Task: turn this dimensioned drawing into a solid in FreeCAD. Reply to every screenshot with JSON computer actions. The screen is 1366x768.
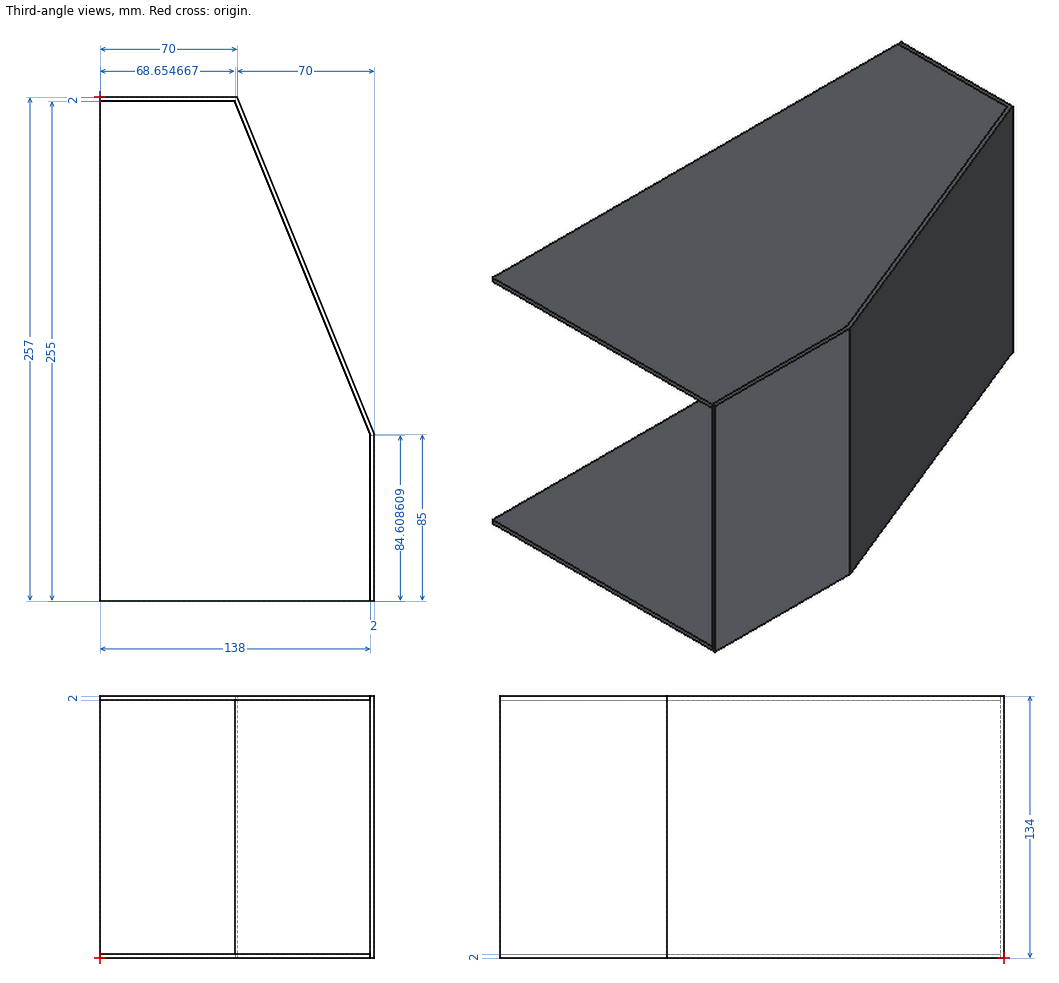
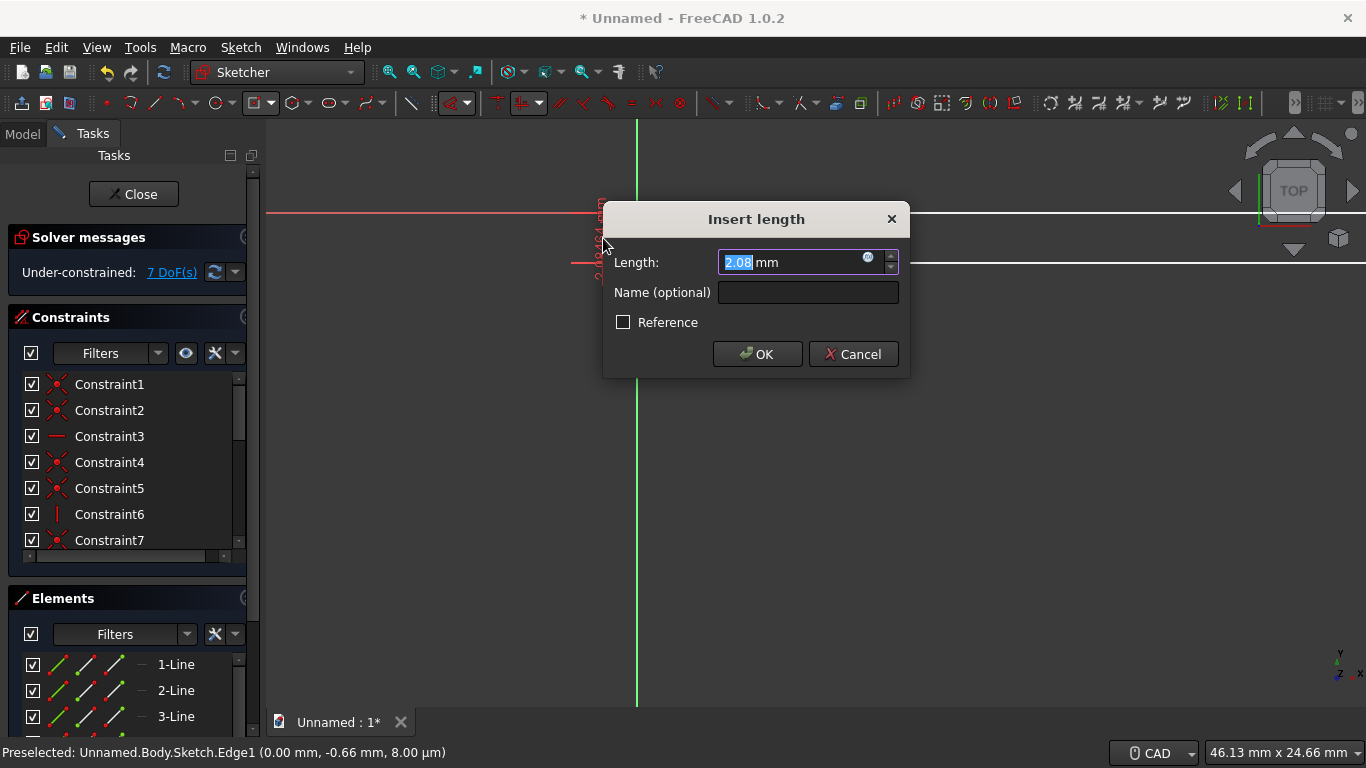
{"action": "type", "text": "2"}
{"action": "key", "text": "Return"}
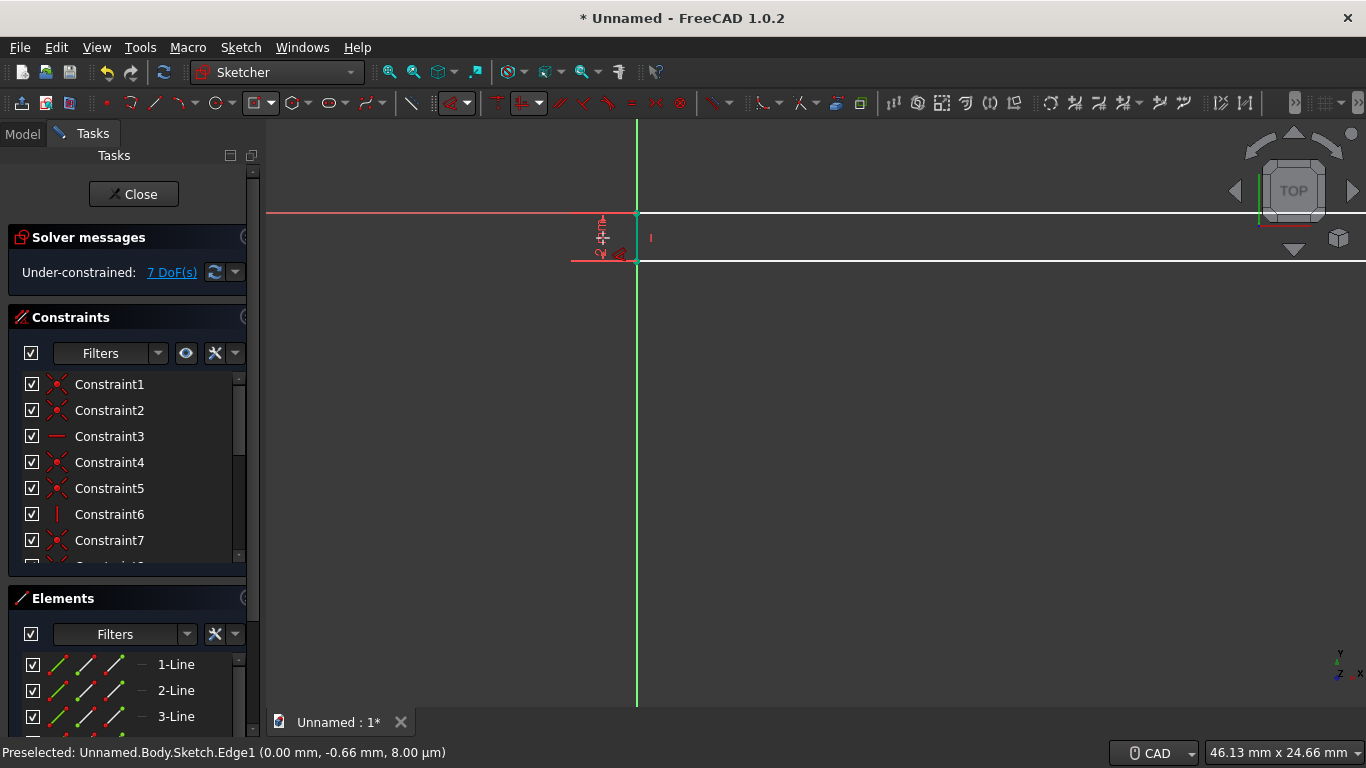
{"action": "scroll", "coordinate": [647, 228], "scroll_direction": "down", "scroll_amount": 14}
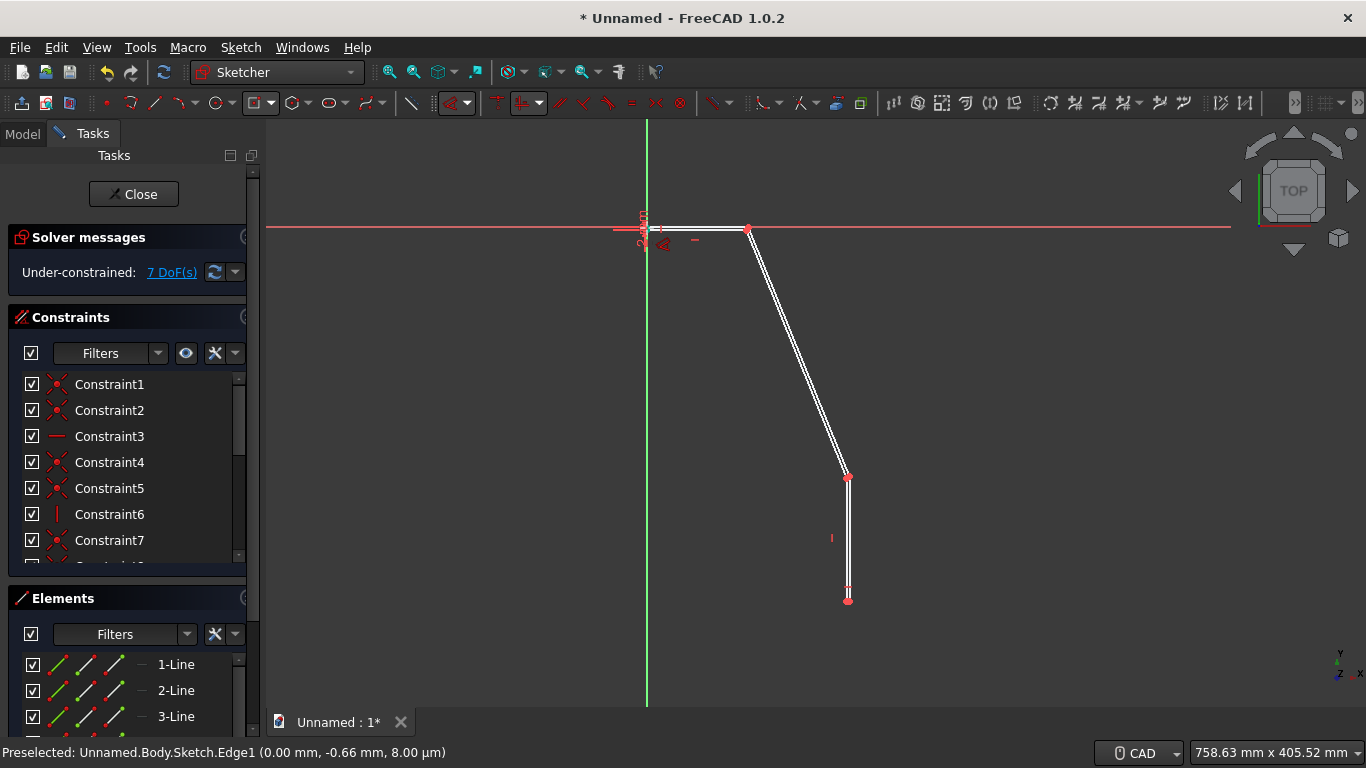
{"action": "scroll", "coordinate": [848, 601], "scroll_direction": "up", "scroll_amount": 14}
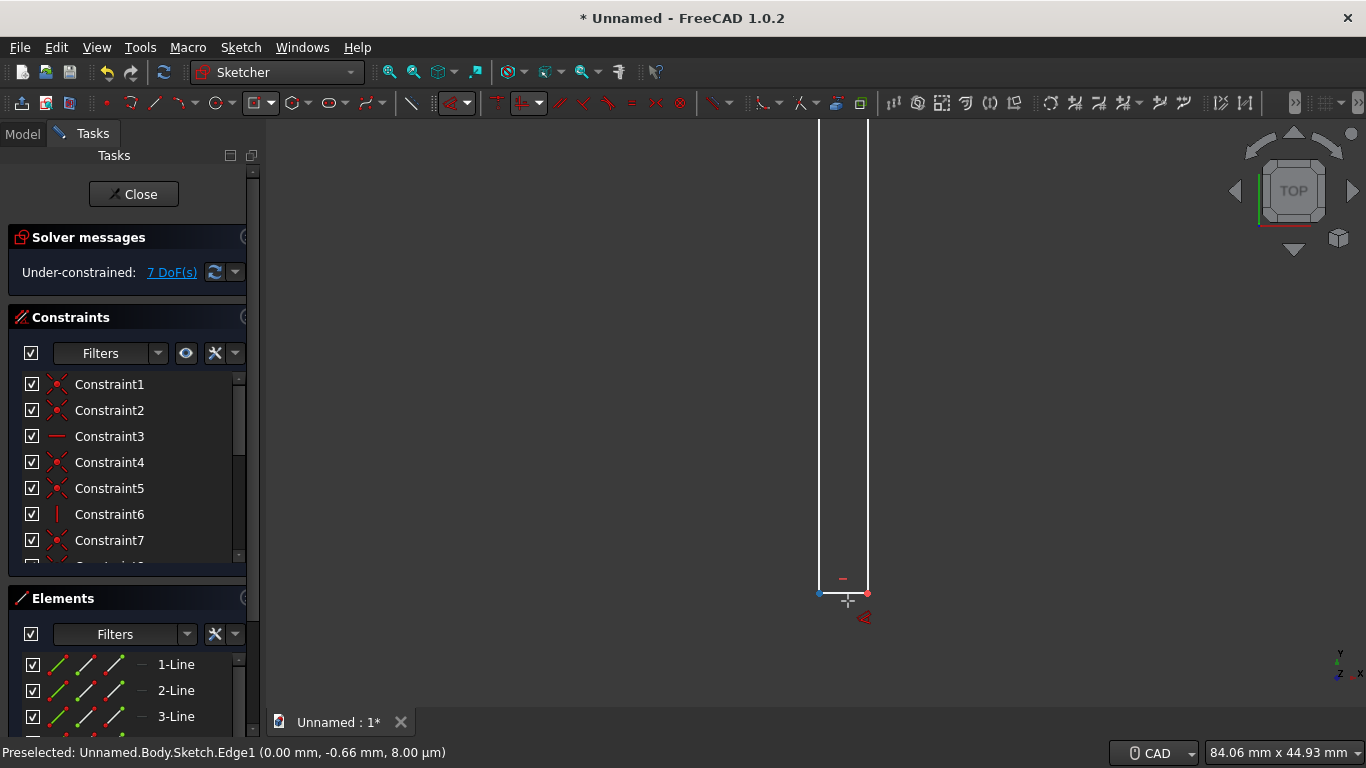
{"action": "left_click", "coordinate": [834, 593]}
{"action": "left_click", "coordinate": [843, 627]}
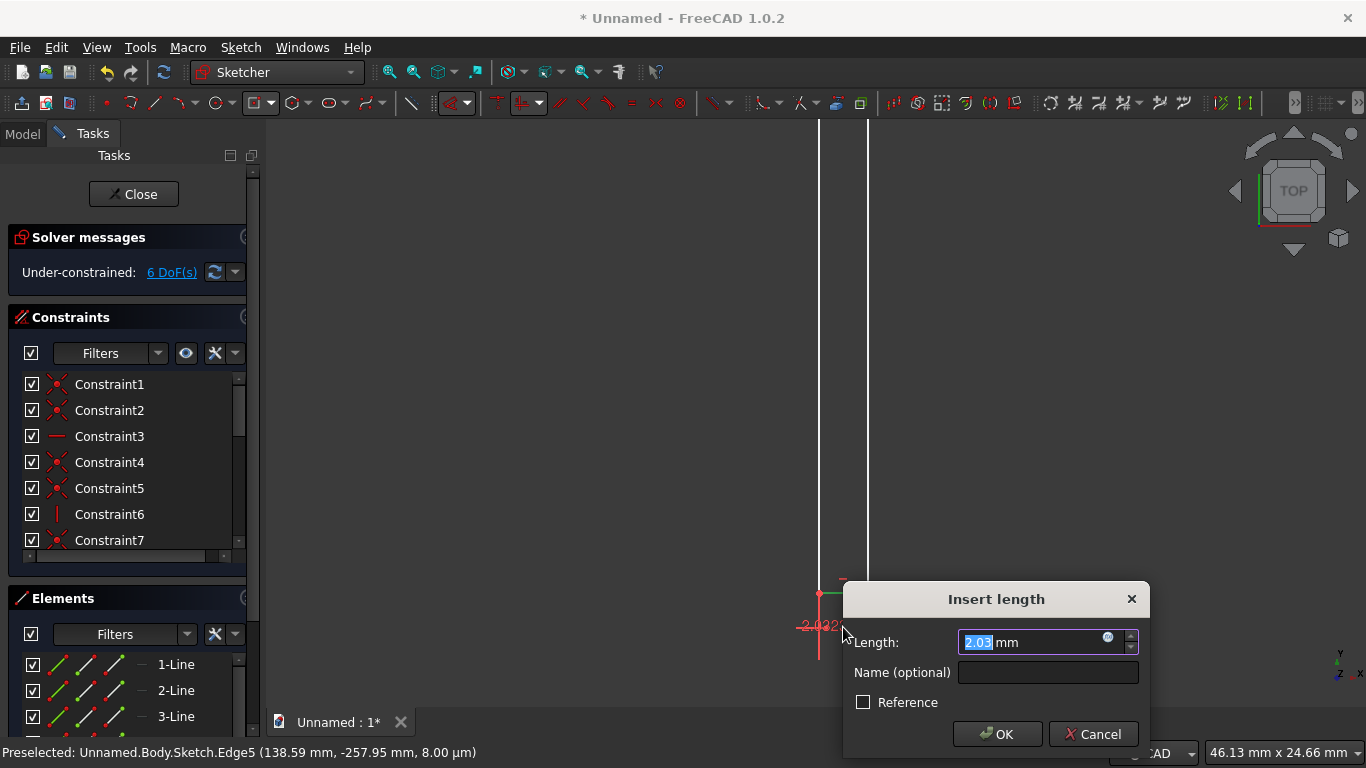
{"action": "type", "text": "2"}
{"action": "key", "text": "Return"}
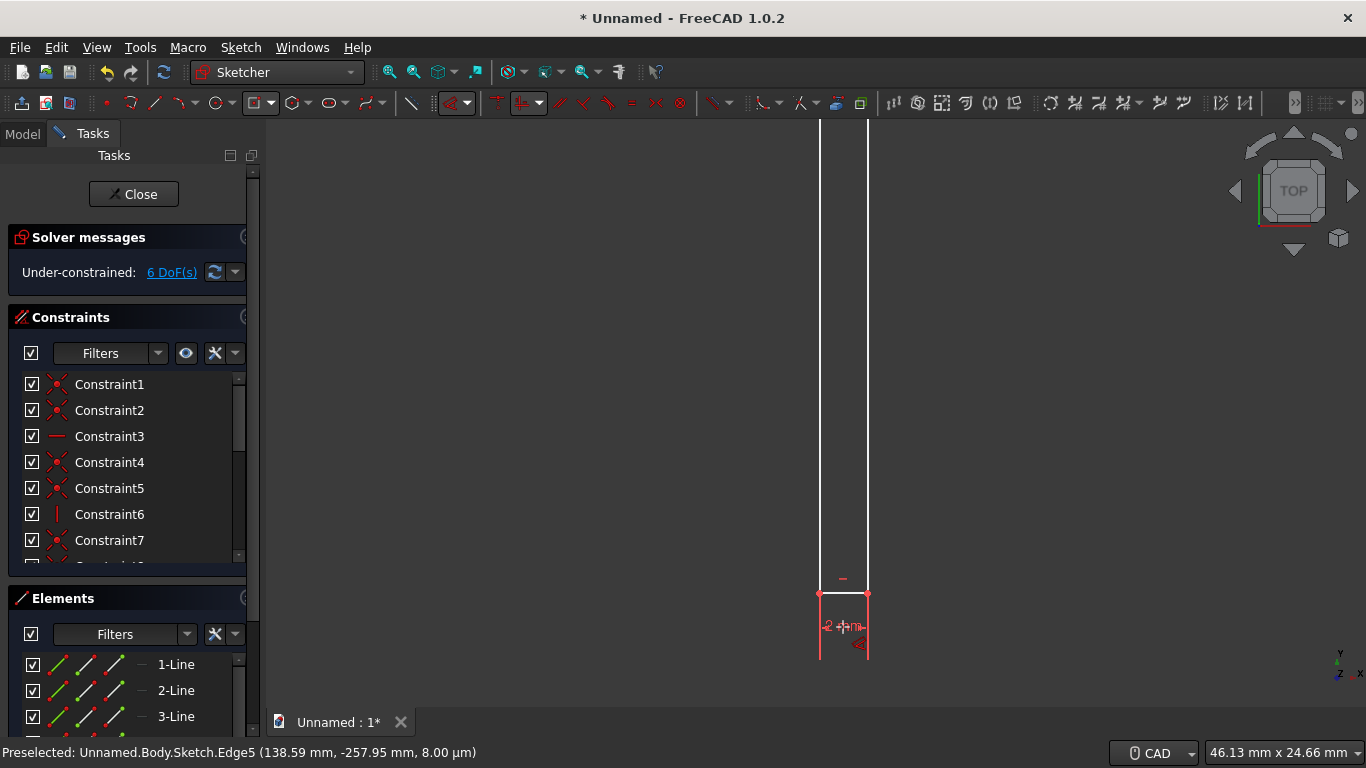
{"action": "scroll", "coordinate": [848, 601], "scroll_direction": "down", "scroll_amount": 14}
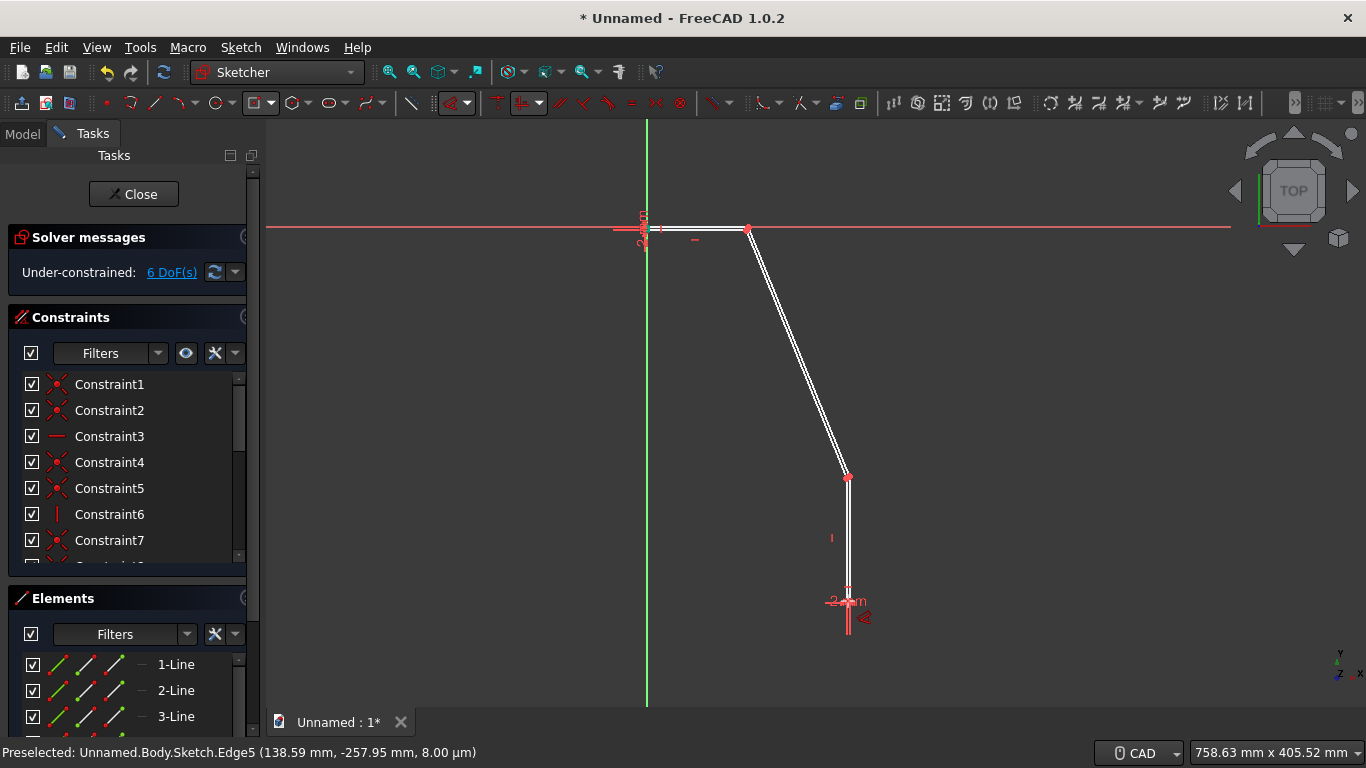
{"action": "scroll", "coordinate": [850, 576], "scroll_direction": "up", "scroll_amount": 8}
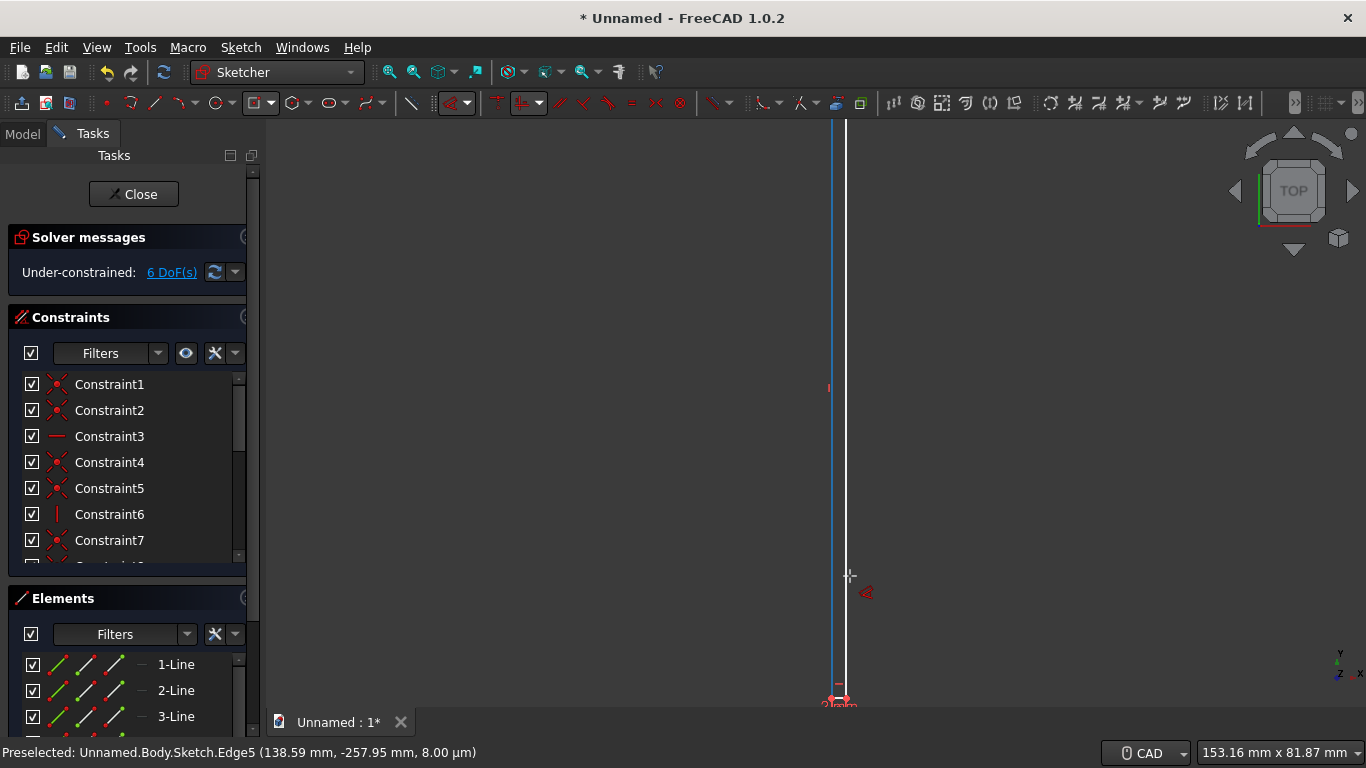
{"action": "left_click", "coordinate": [846, 575]}
{"action": "left_click", "coordinate": [880, 413]}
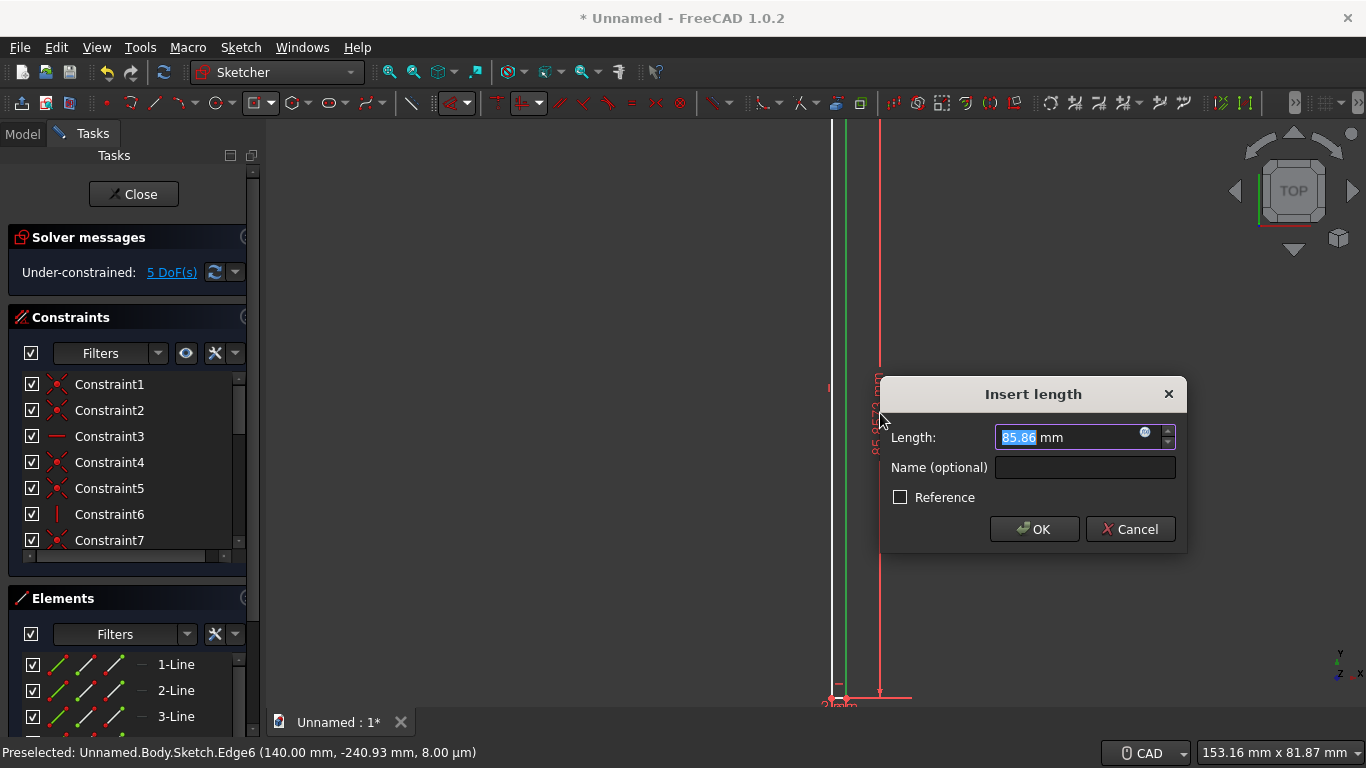
{"action": "type", "text": "85"}
{"action": "key", "text": "Return"}